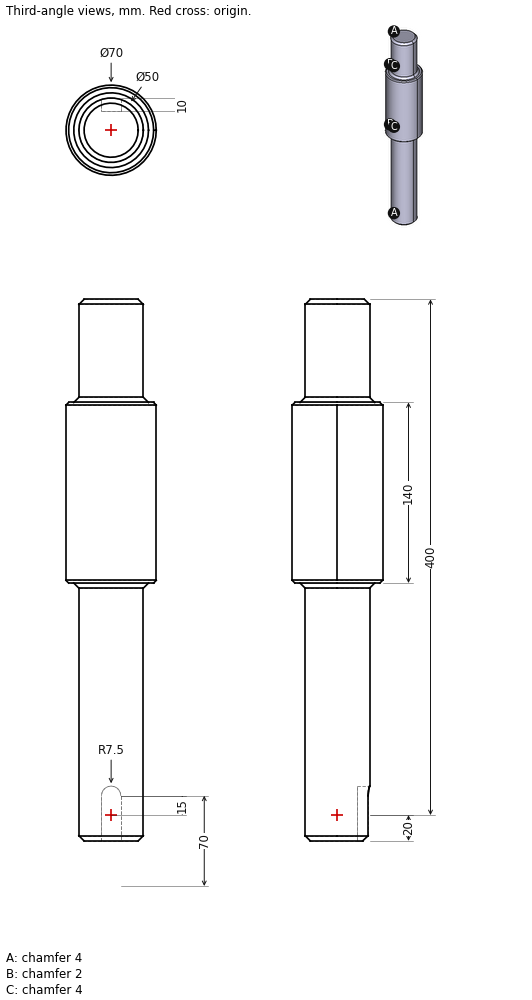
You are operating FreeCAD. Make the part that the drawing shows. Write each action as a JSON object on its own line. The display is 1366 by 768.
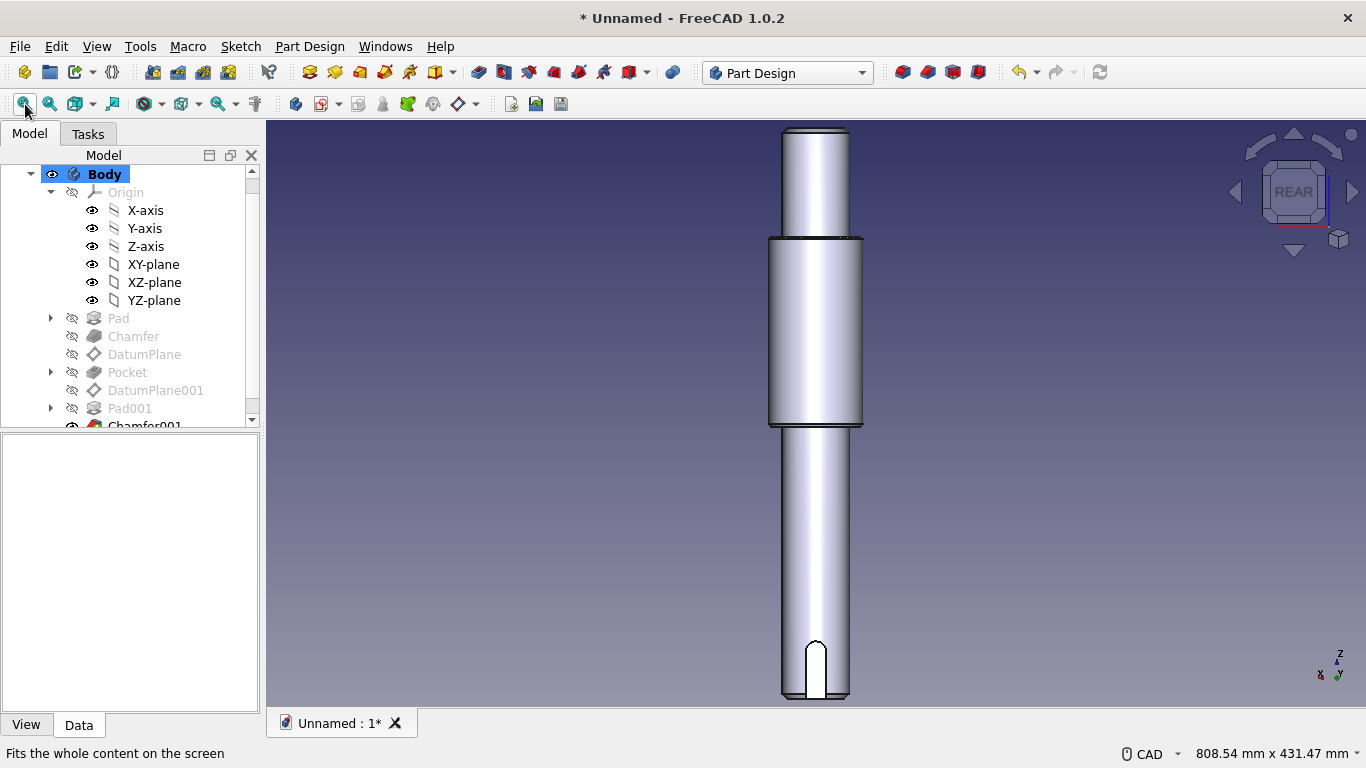
{"action": "key", "text": "6"}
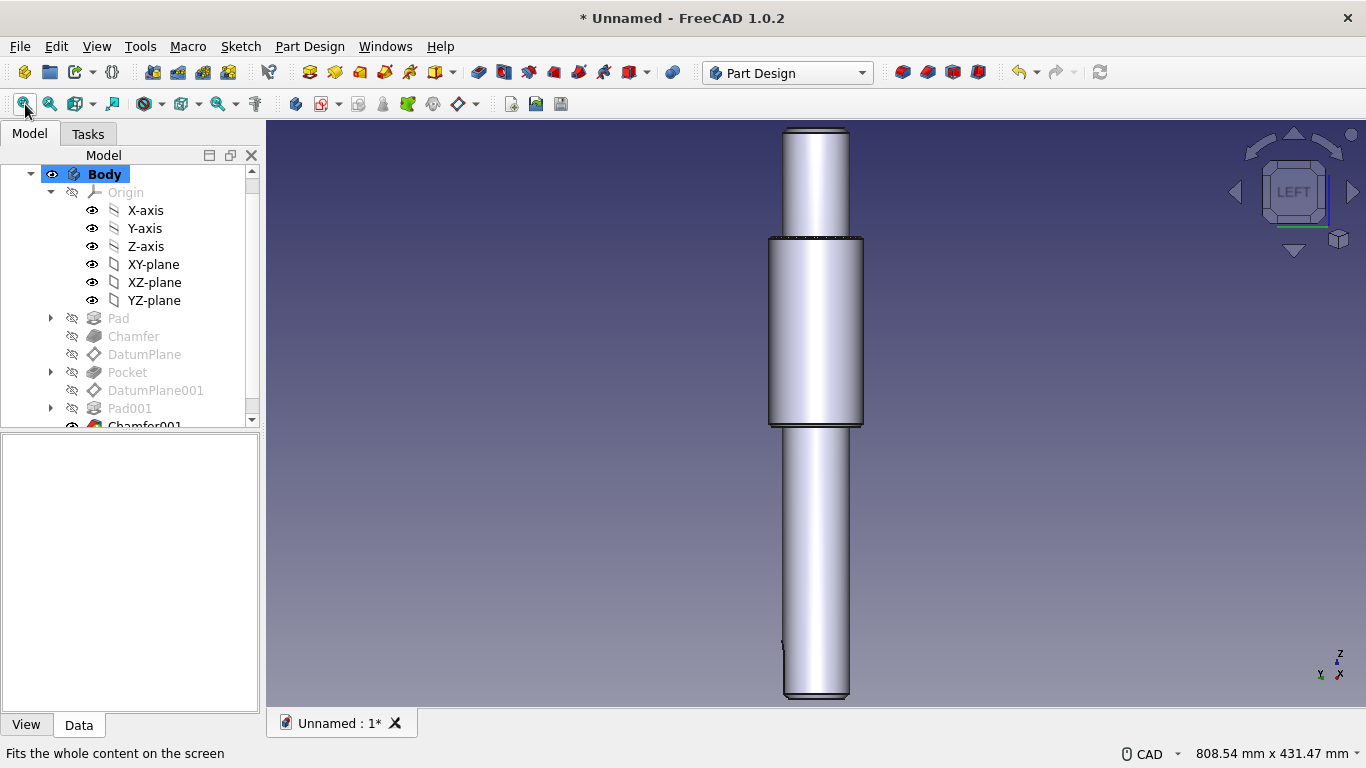
{"action": "key", "text": "v 3"}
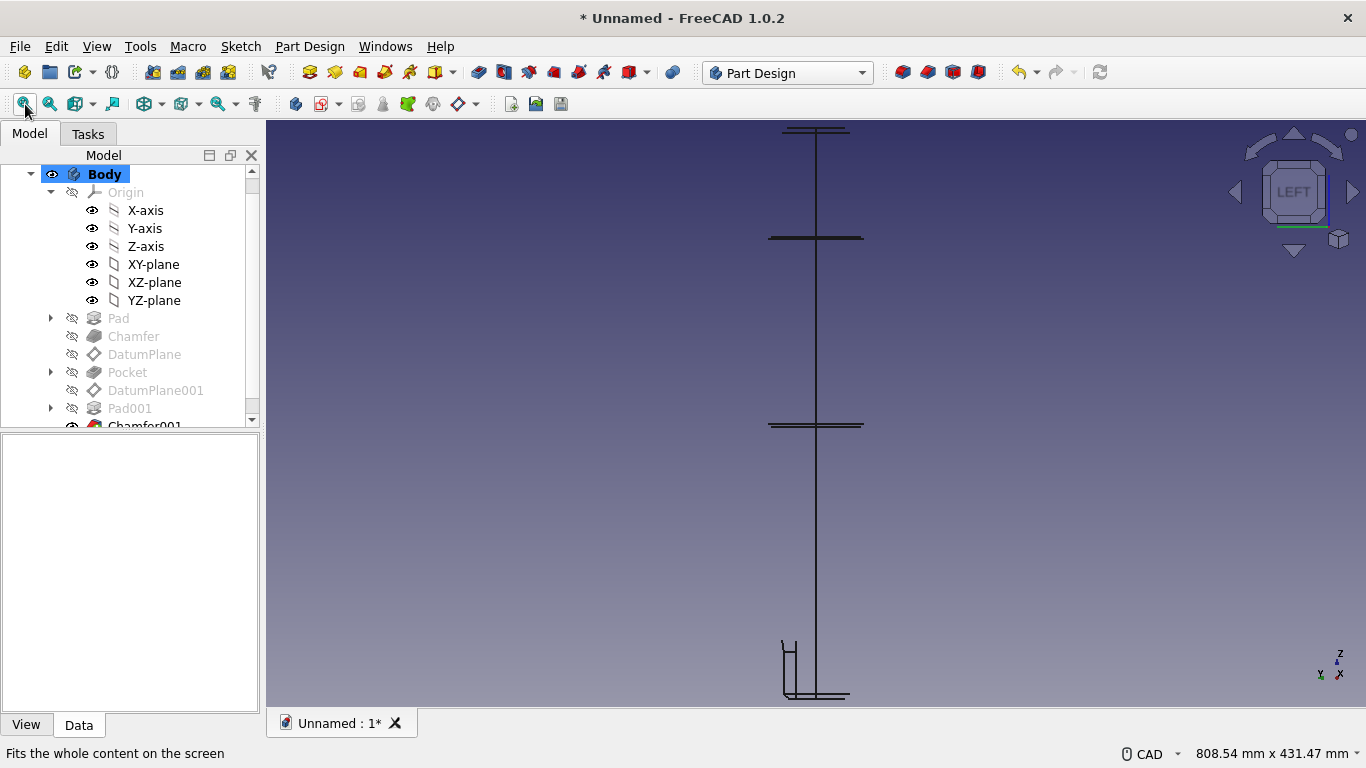
{"action": "key", "text": "0"}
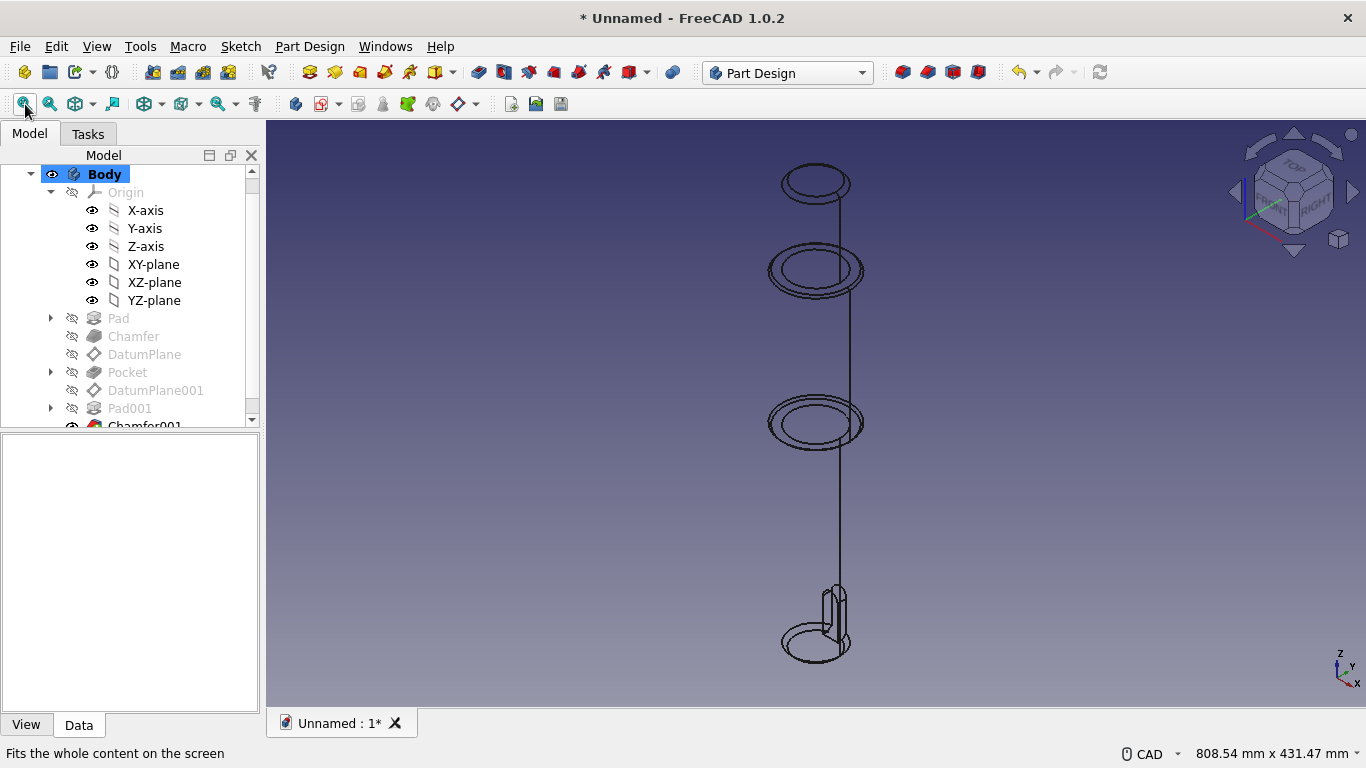
{"action": "left_click", "coordinate": [792, 254]}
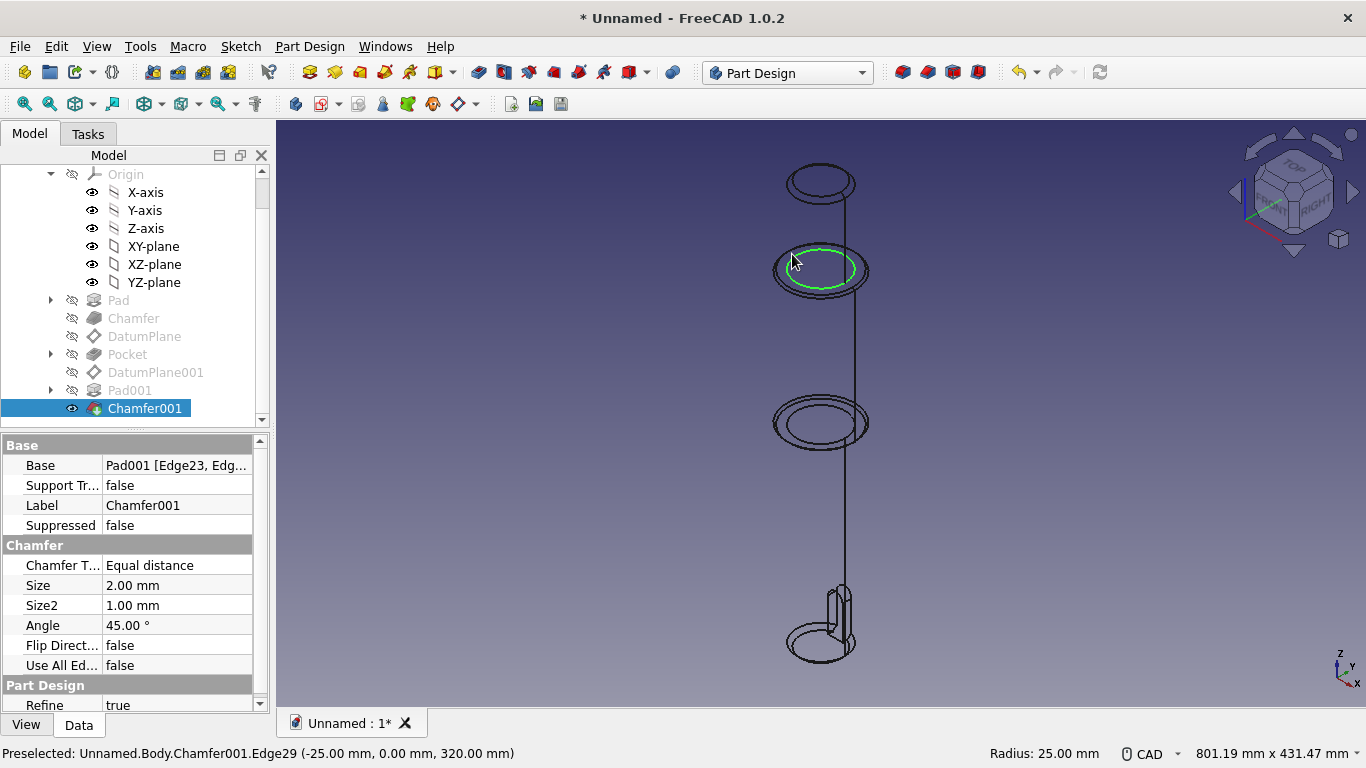
{"action": "left_click", "coordinate": [797, 410], "text": "ctrl"}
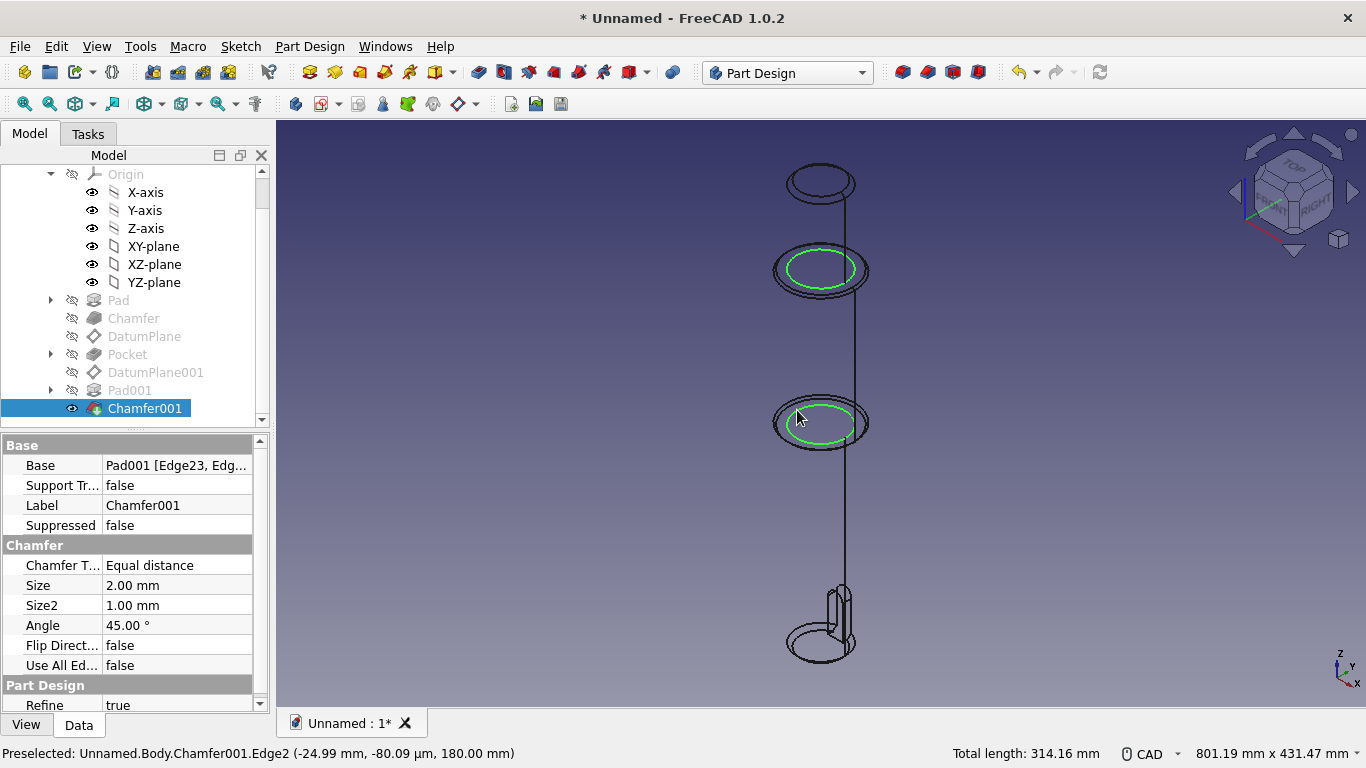
{"action": "key", "text": "v 1"}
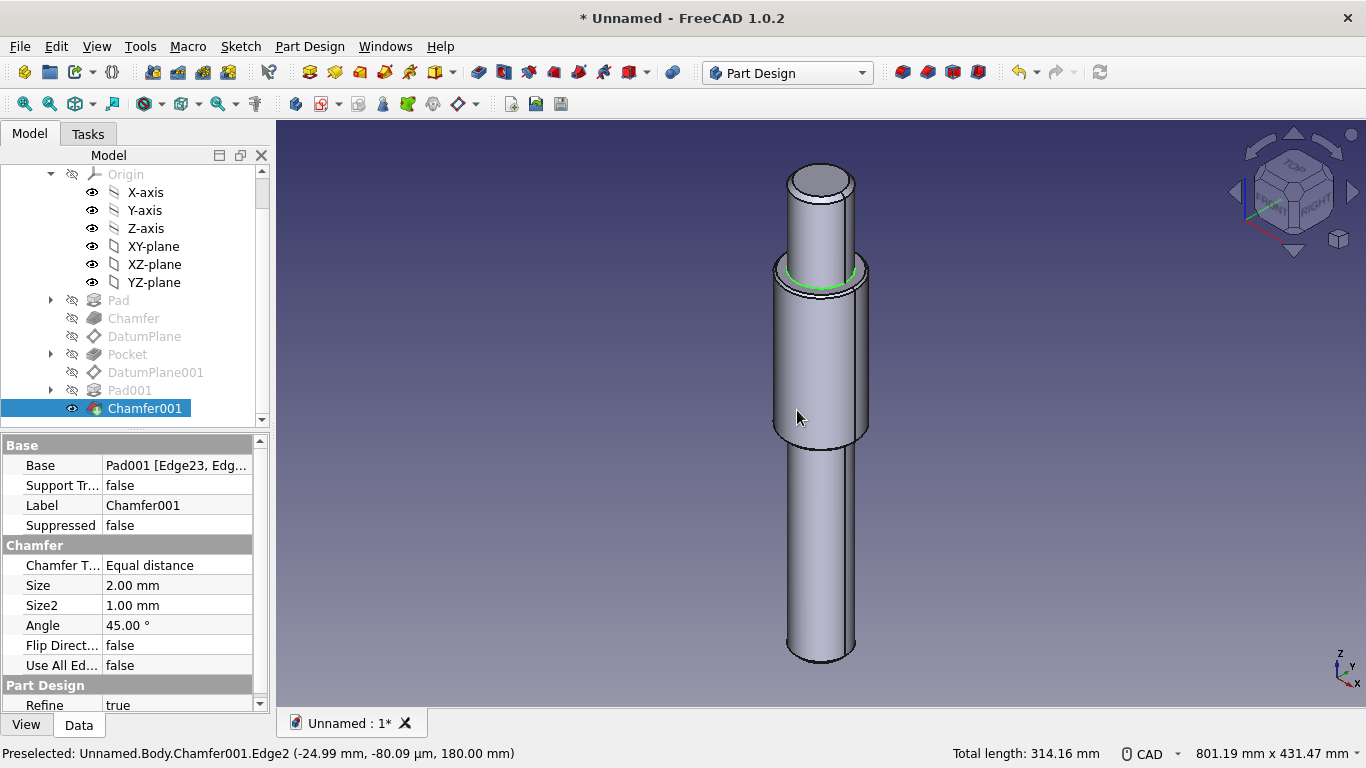
{"action": "left_click", "coordinate": [928, 72]}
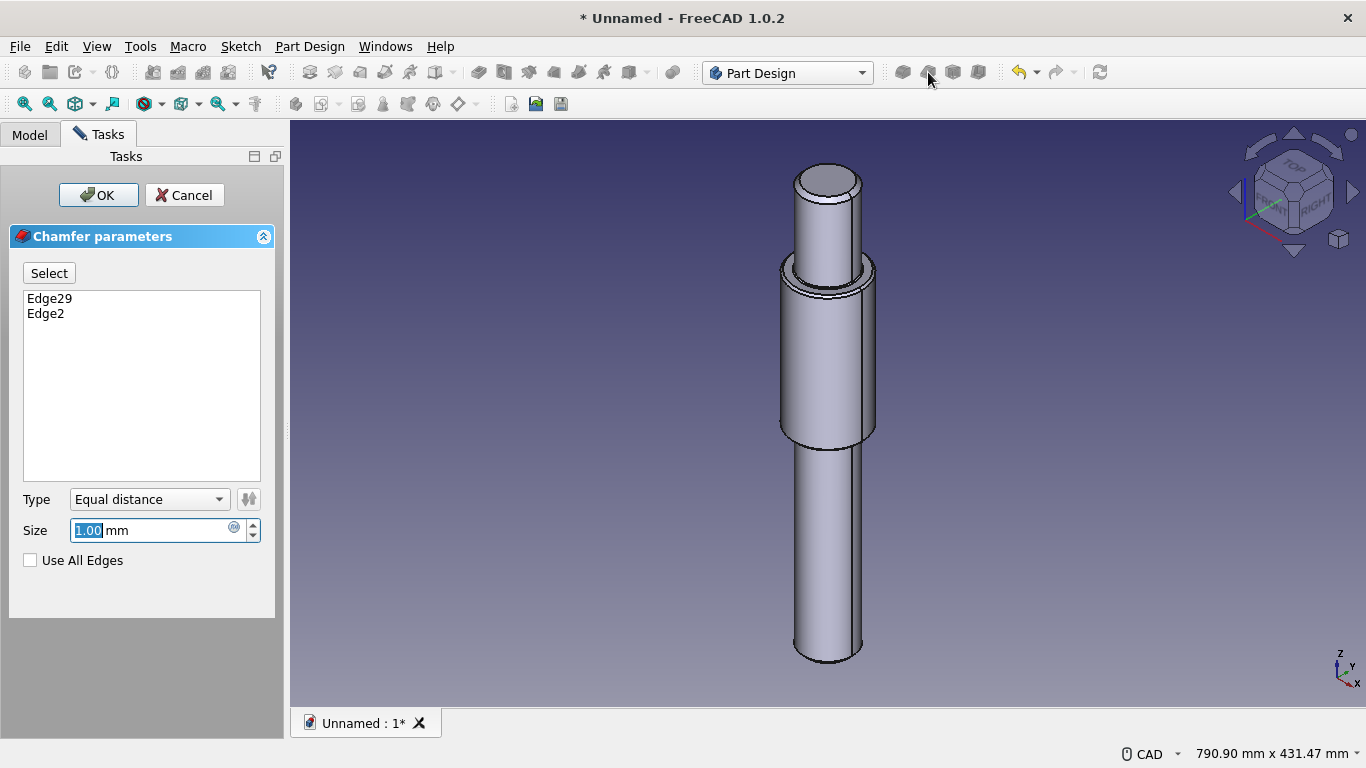
{"action": "type", "text": "4"}
{"action": "key", "text": "Tab"}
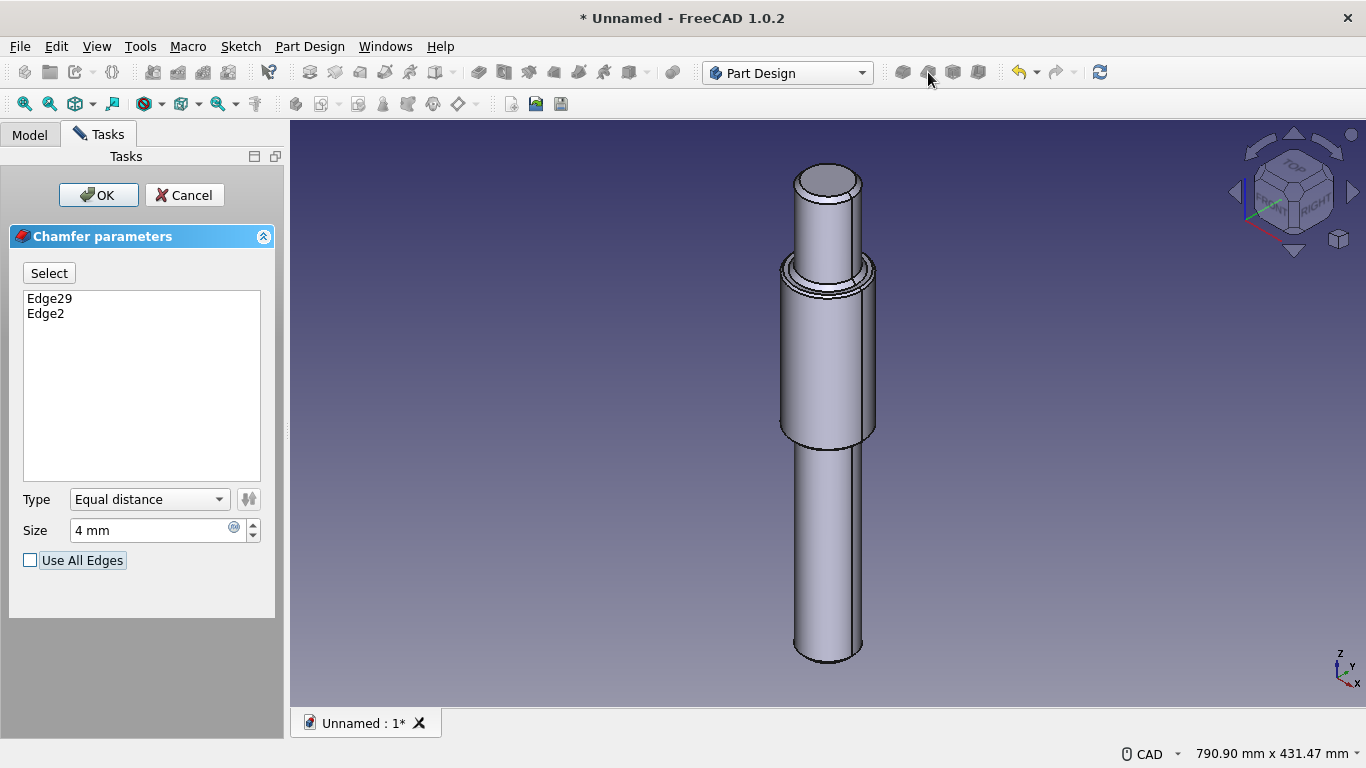
{"action": "left_click", "coordinate": [99, 195]}